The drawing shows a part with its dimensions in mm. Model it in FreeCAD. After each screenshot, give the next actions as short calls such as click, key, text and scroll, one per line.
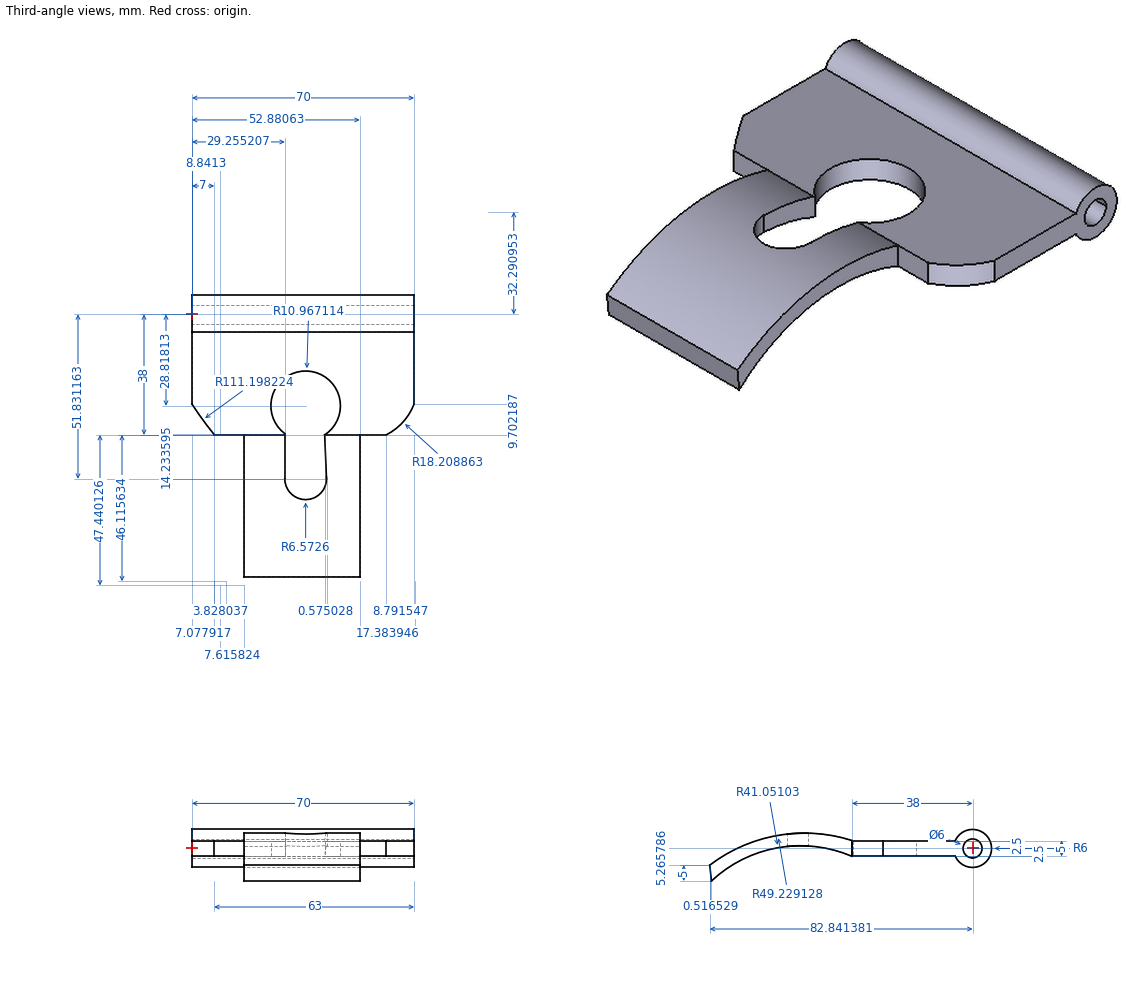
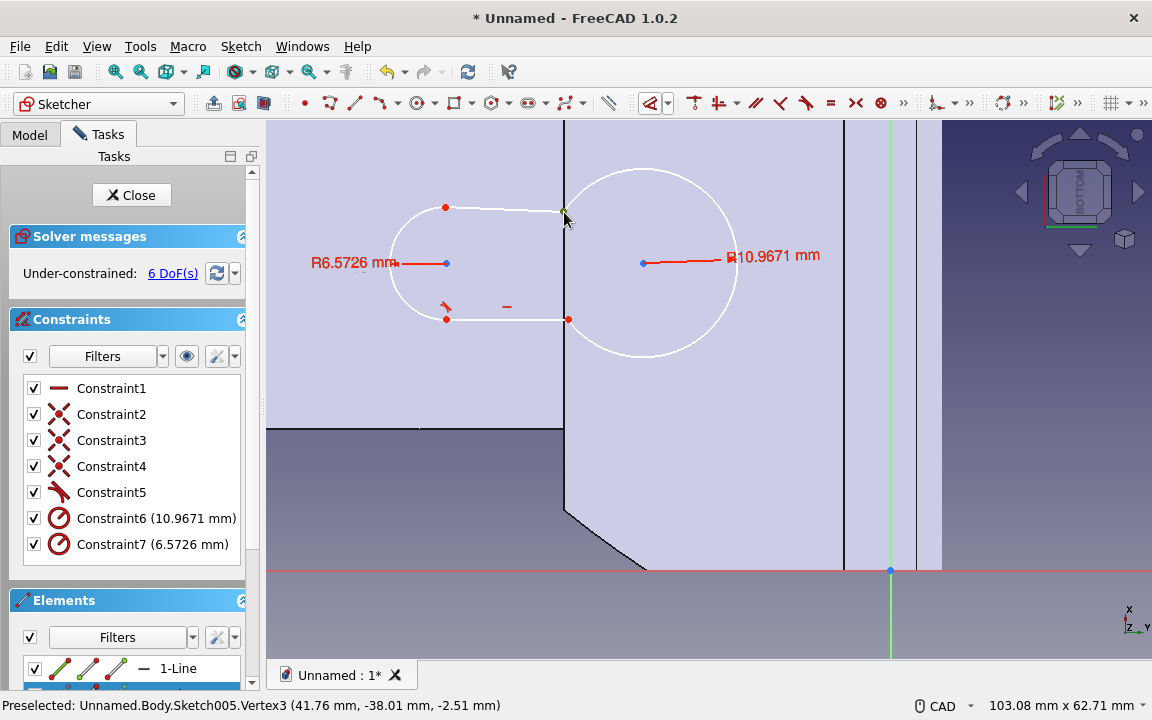
click(668, 104)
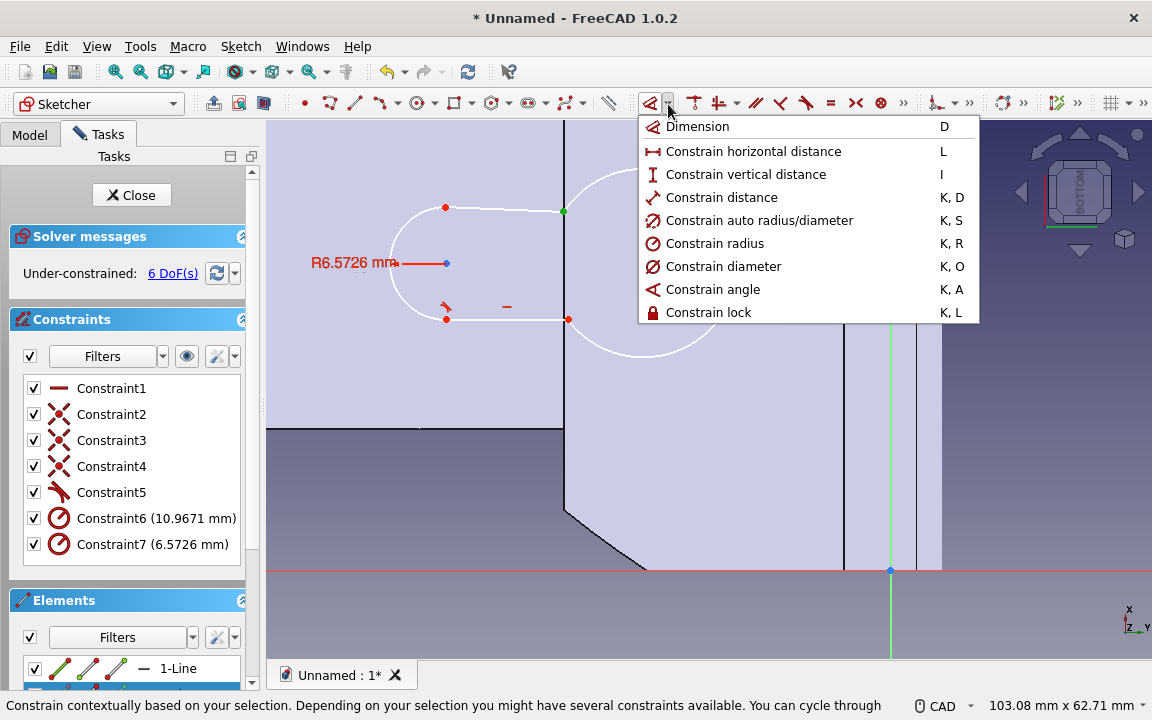
click(809, 152)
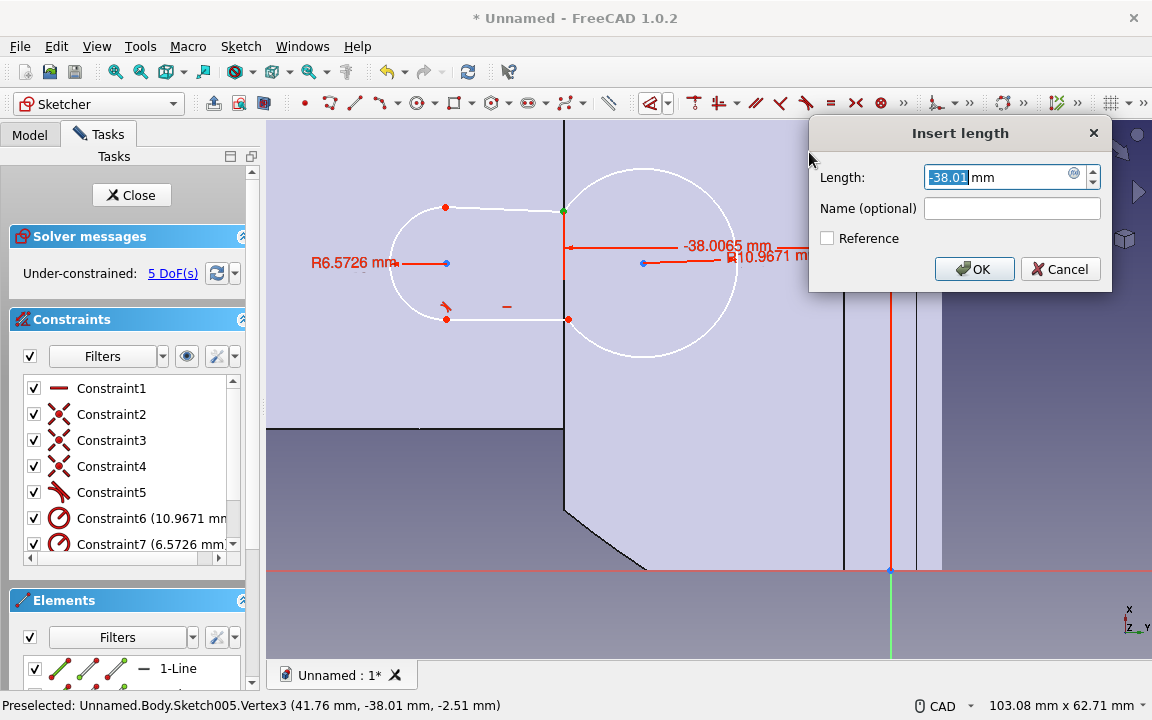
text(-38)
key(Return)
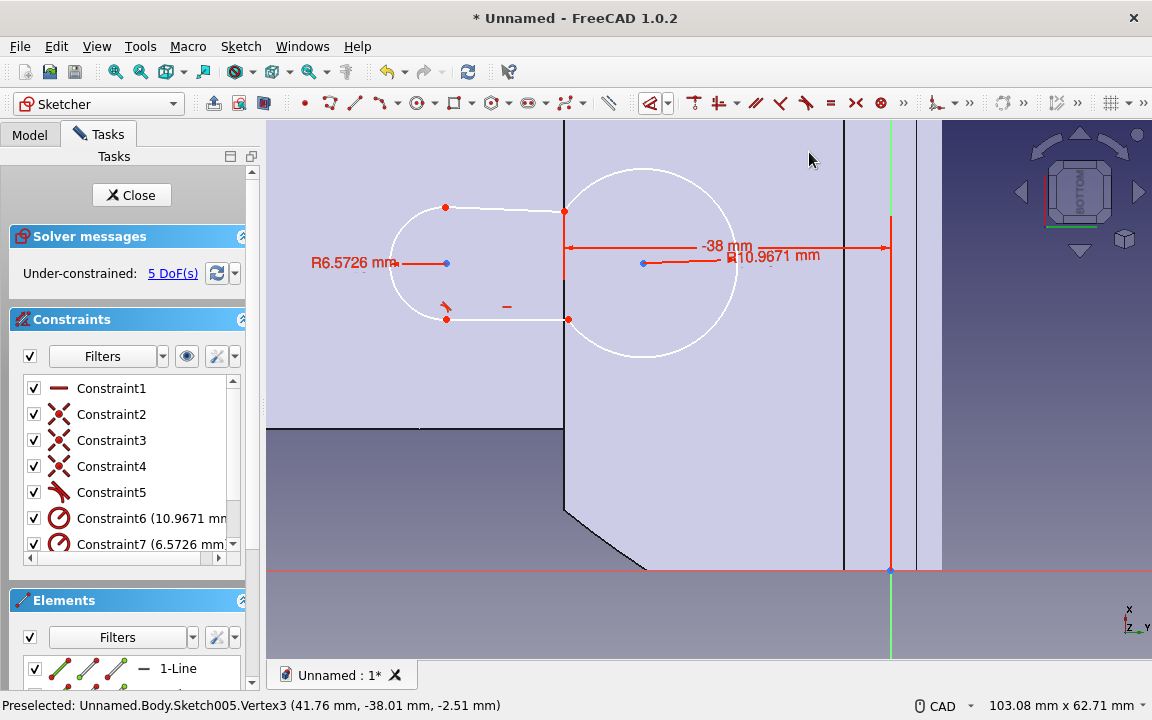
click(483, 320)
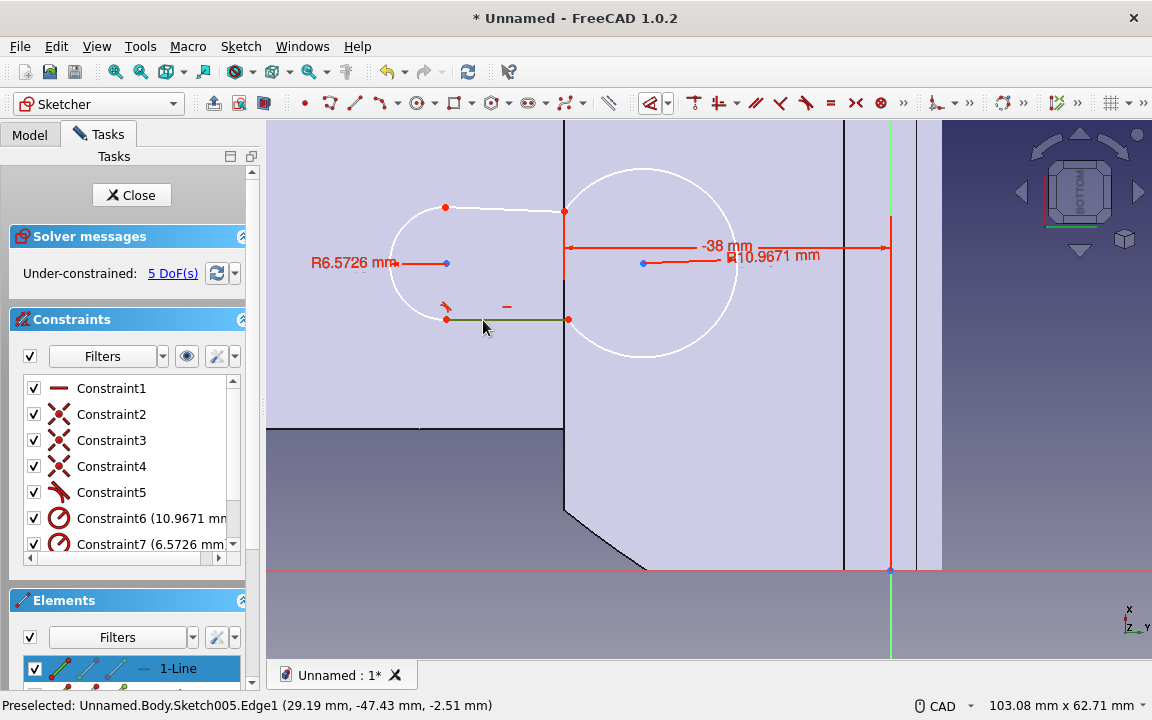
click(668, 104)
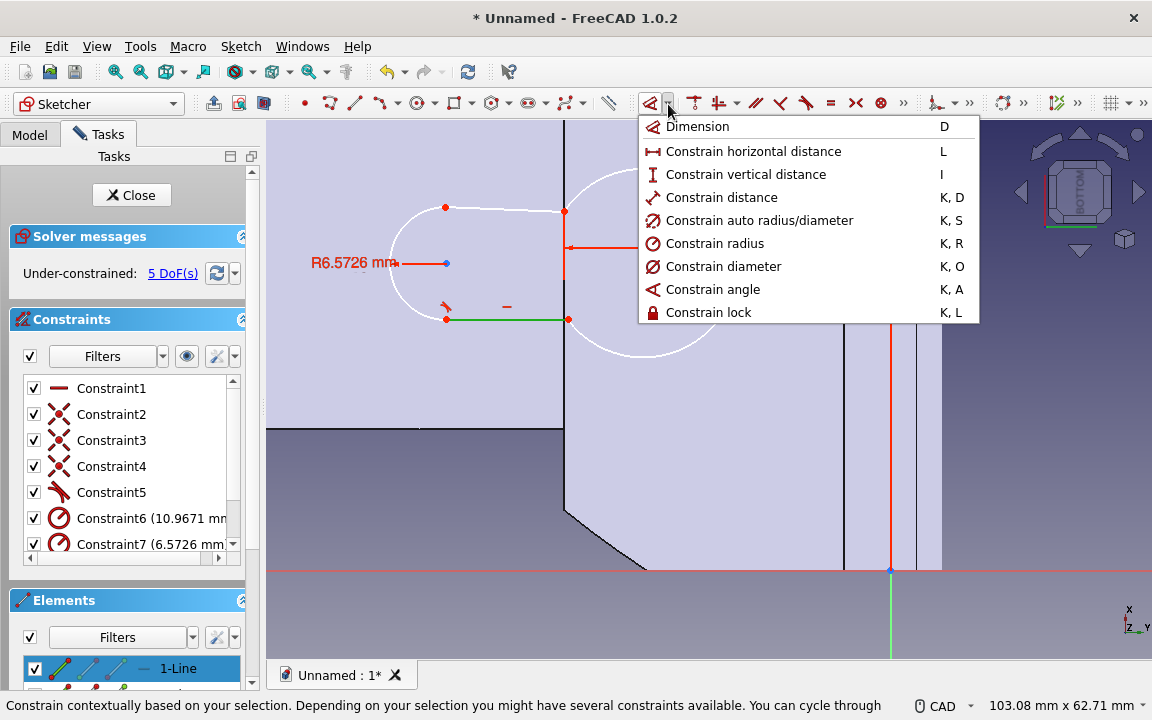
click(809, 152)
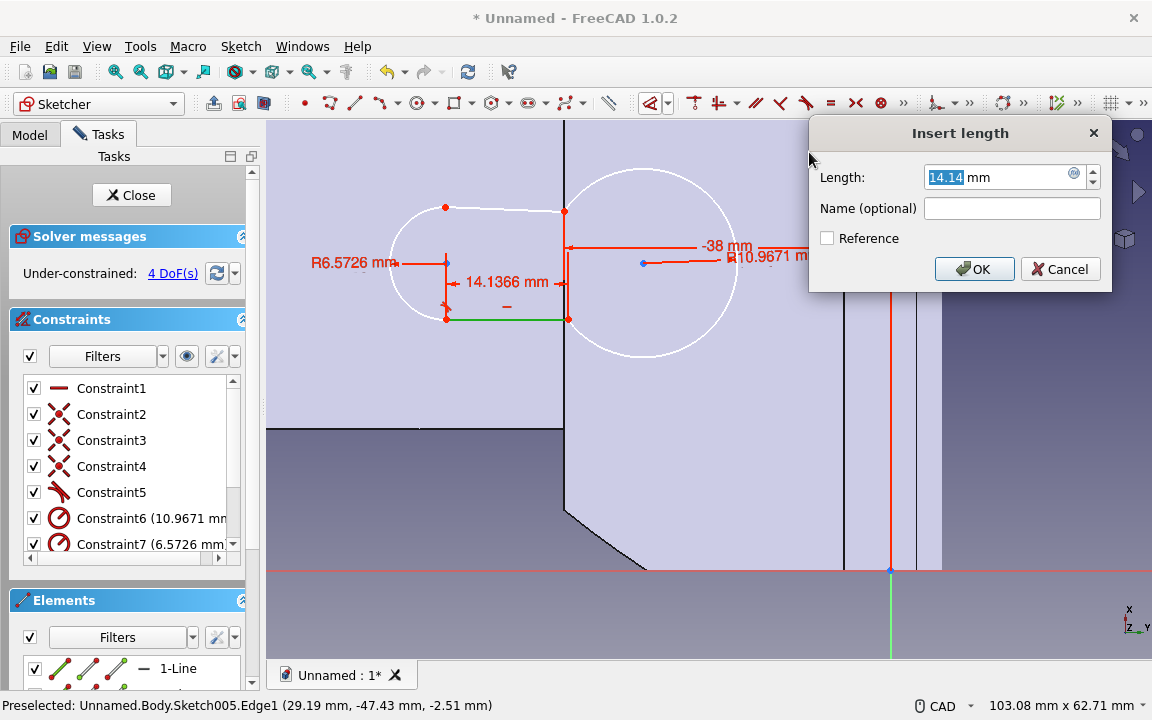
text(14.233595)
key(Return)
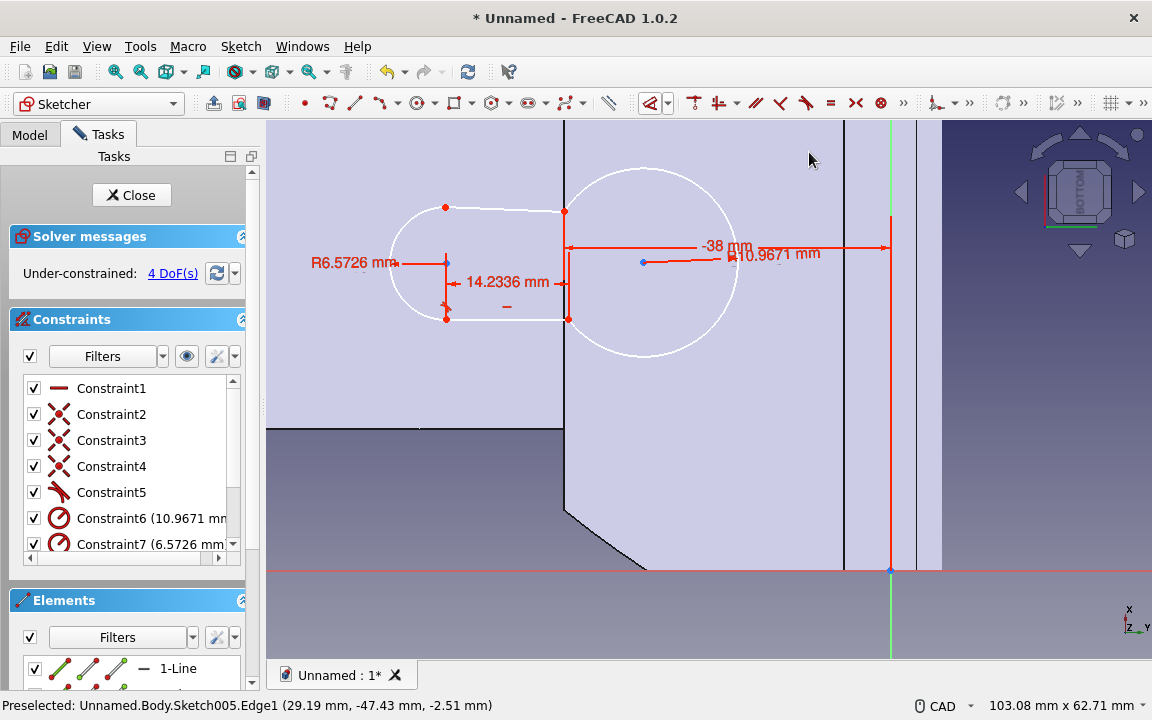
scroll(528, 211, up, 11)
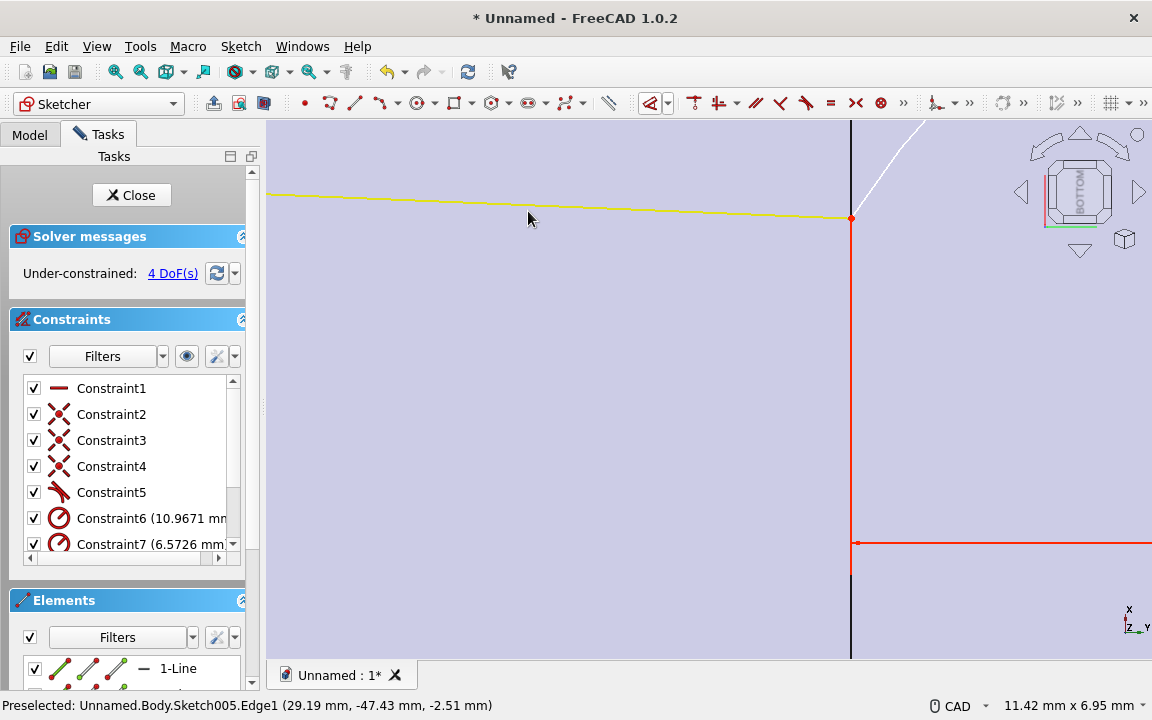
click(529, 205)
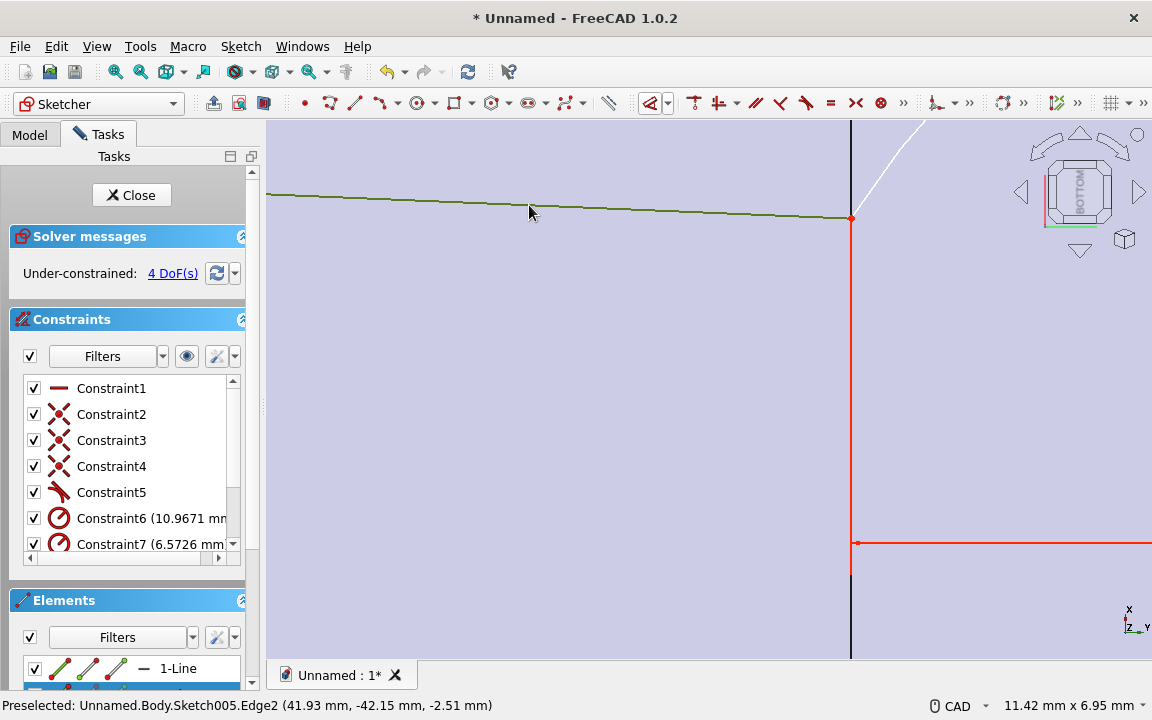
key(i)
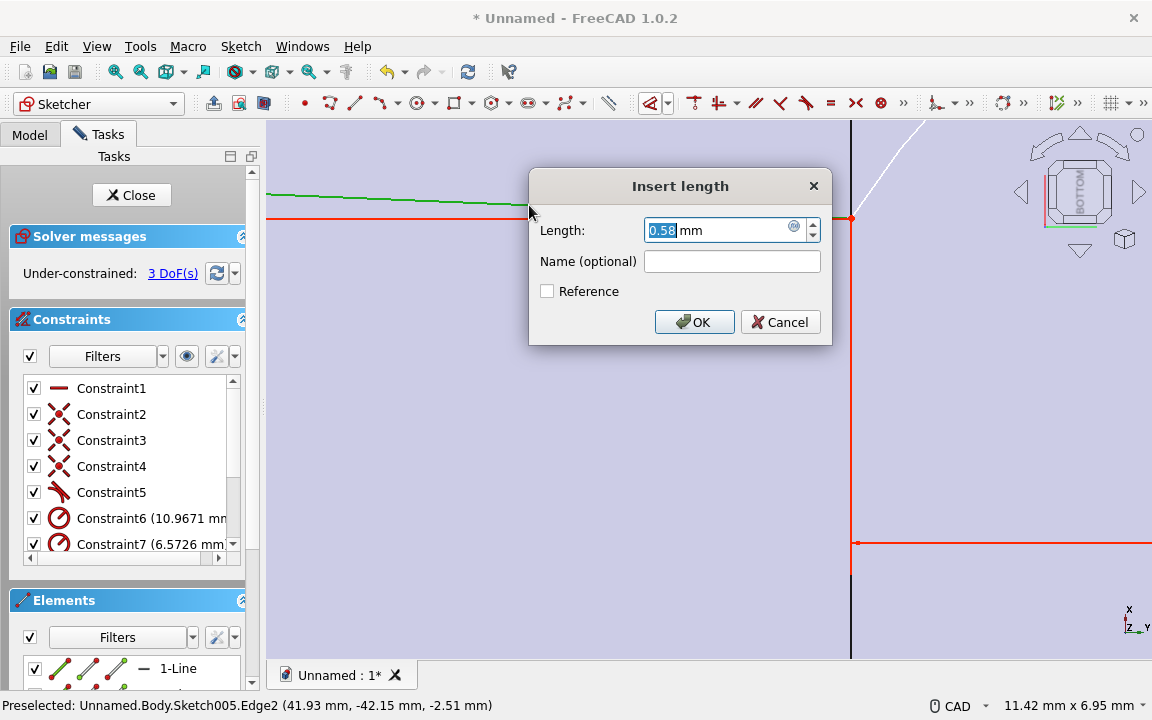
text(0.575028)
key(Return)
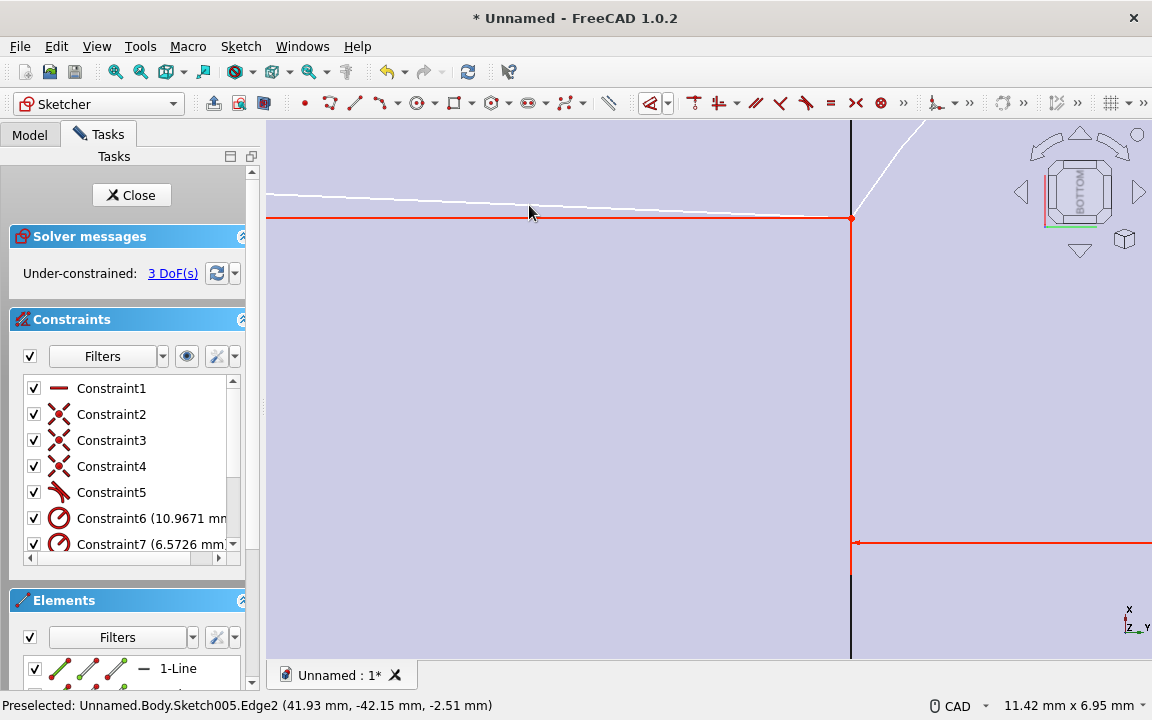
scroll(529, 212, down, 11)